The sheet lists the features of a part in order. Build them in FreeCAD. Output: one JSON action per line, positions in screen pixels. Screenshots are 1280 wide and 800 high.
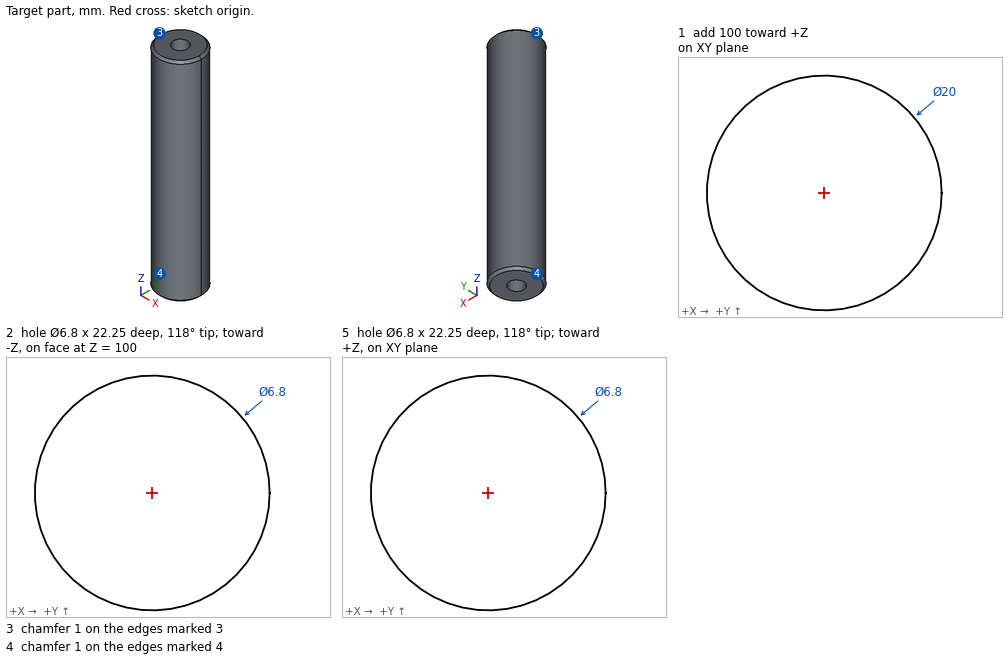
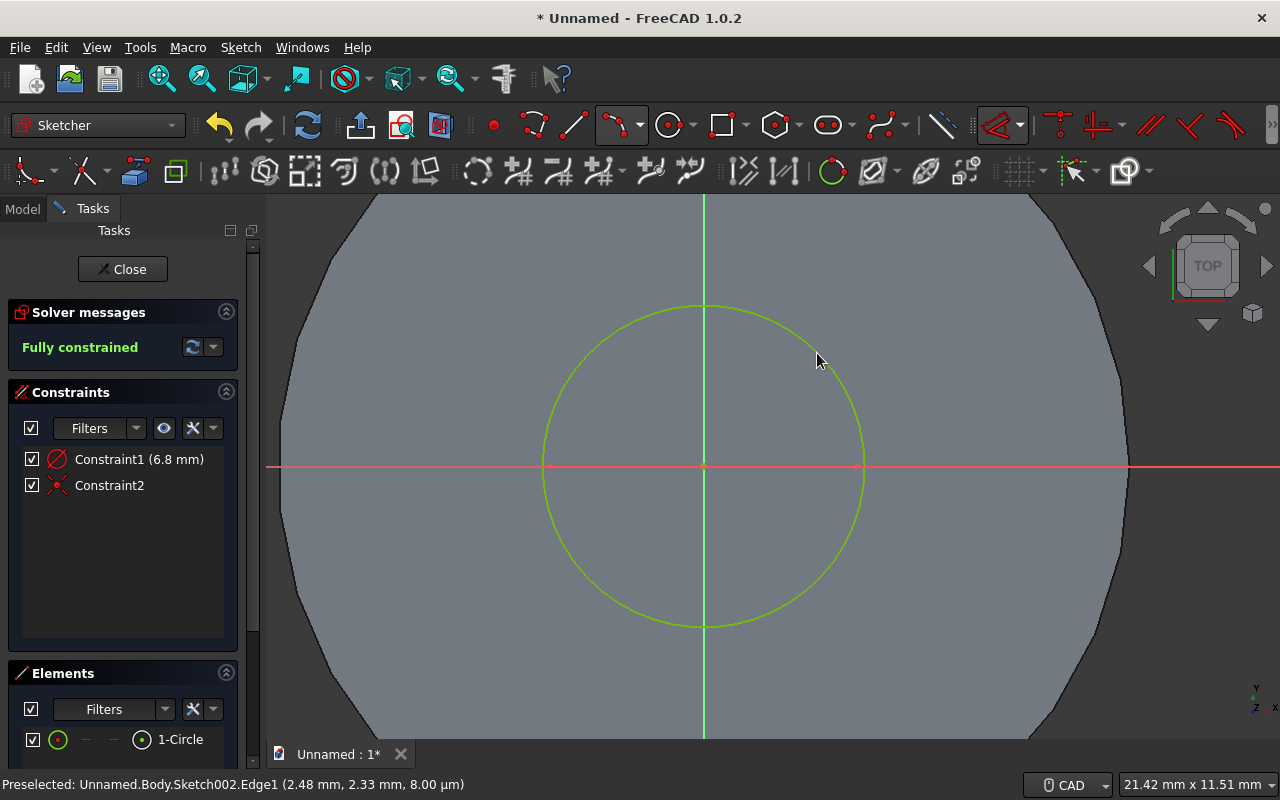
{"action": "left_click", "coordinate": [123, 269]}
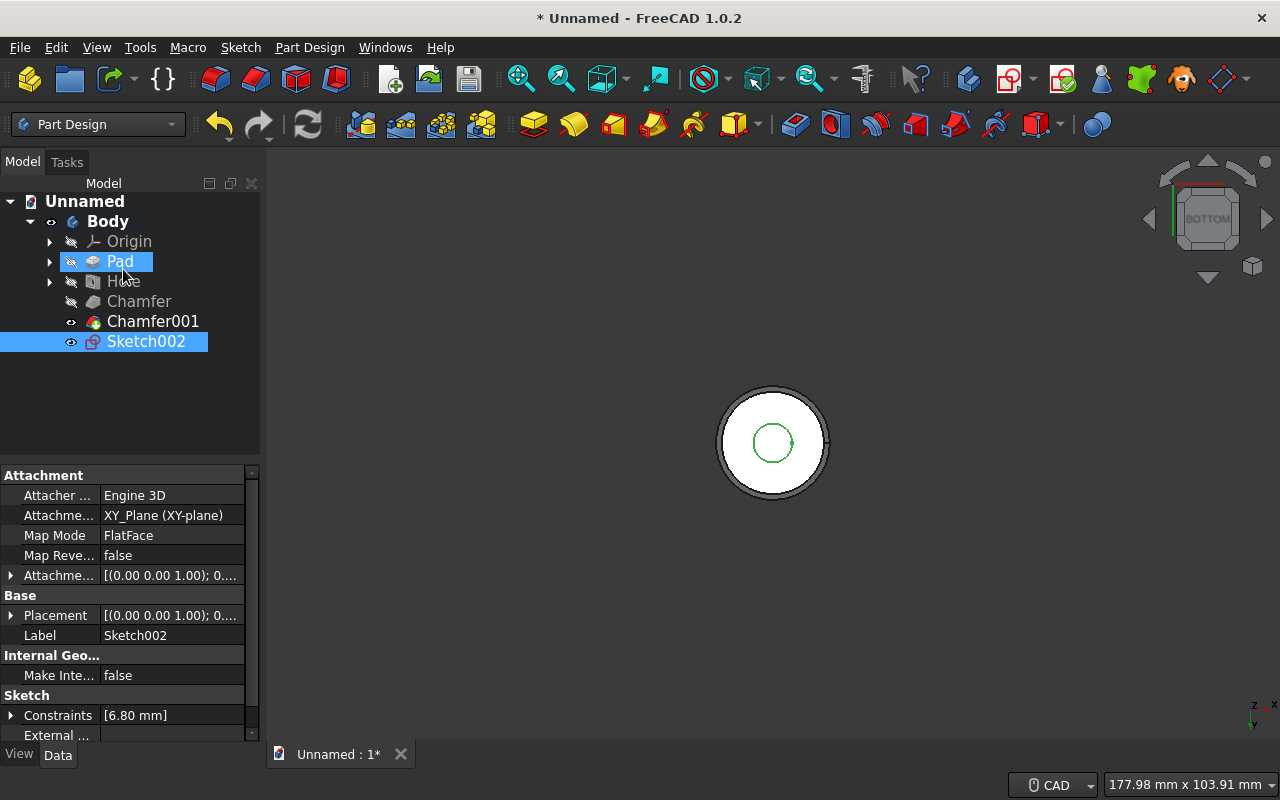
{"action": "left_click", "coordinate": [836, 124]}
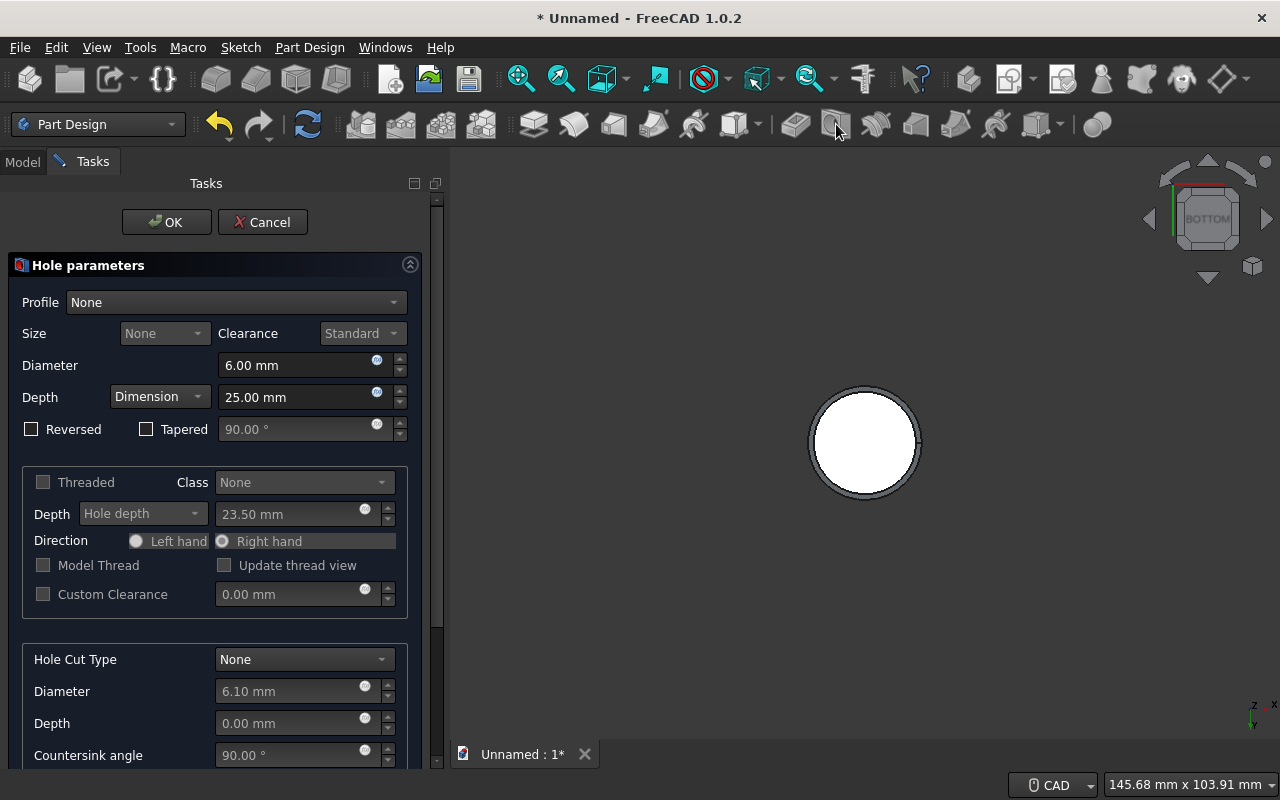
{"action": "triple_click", "coordinate": [305, 365]}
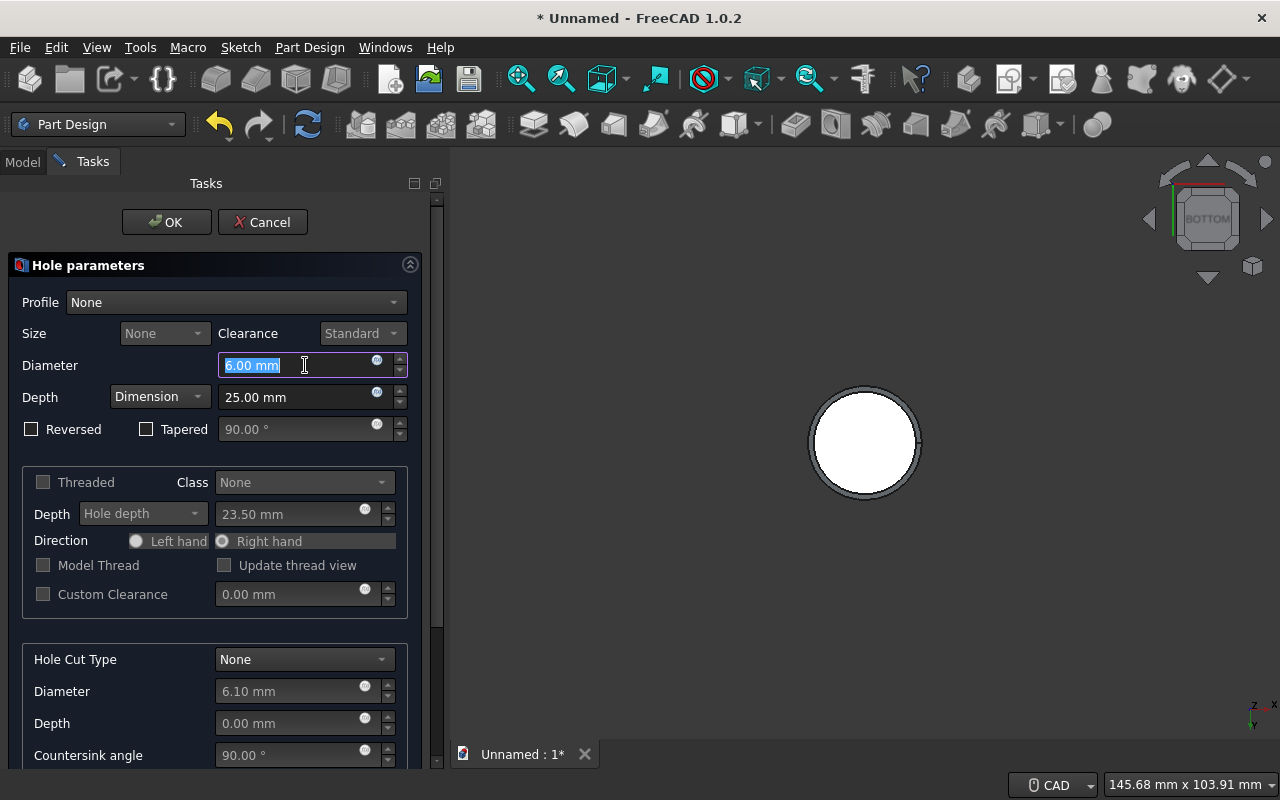
{"action": "type", "text": "6.8"}
{"action": "key", "text": "Tab"}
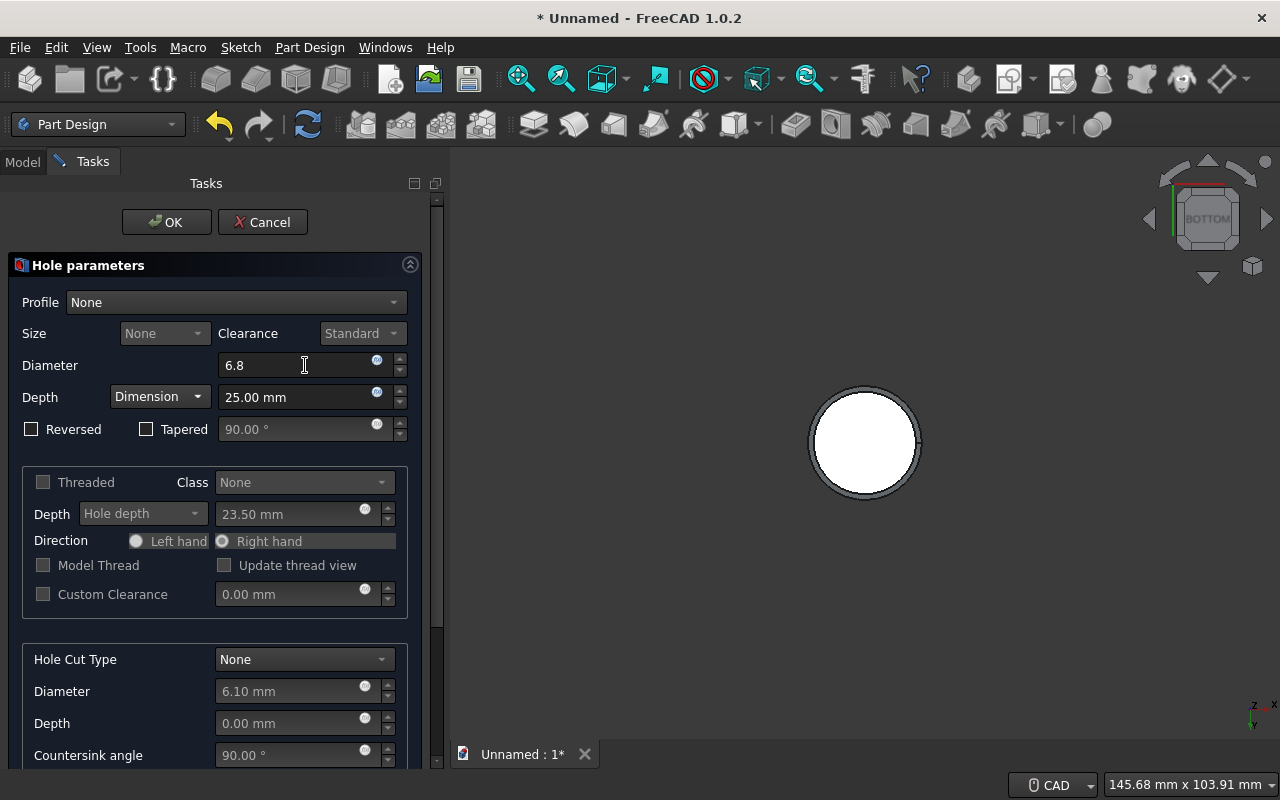
{"action": "triple_click", "coordinate": [305, 397]}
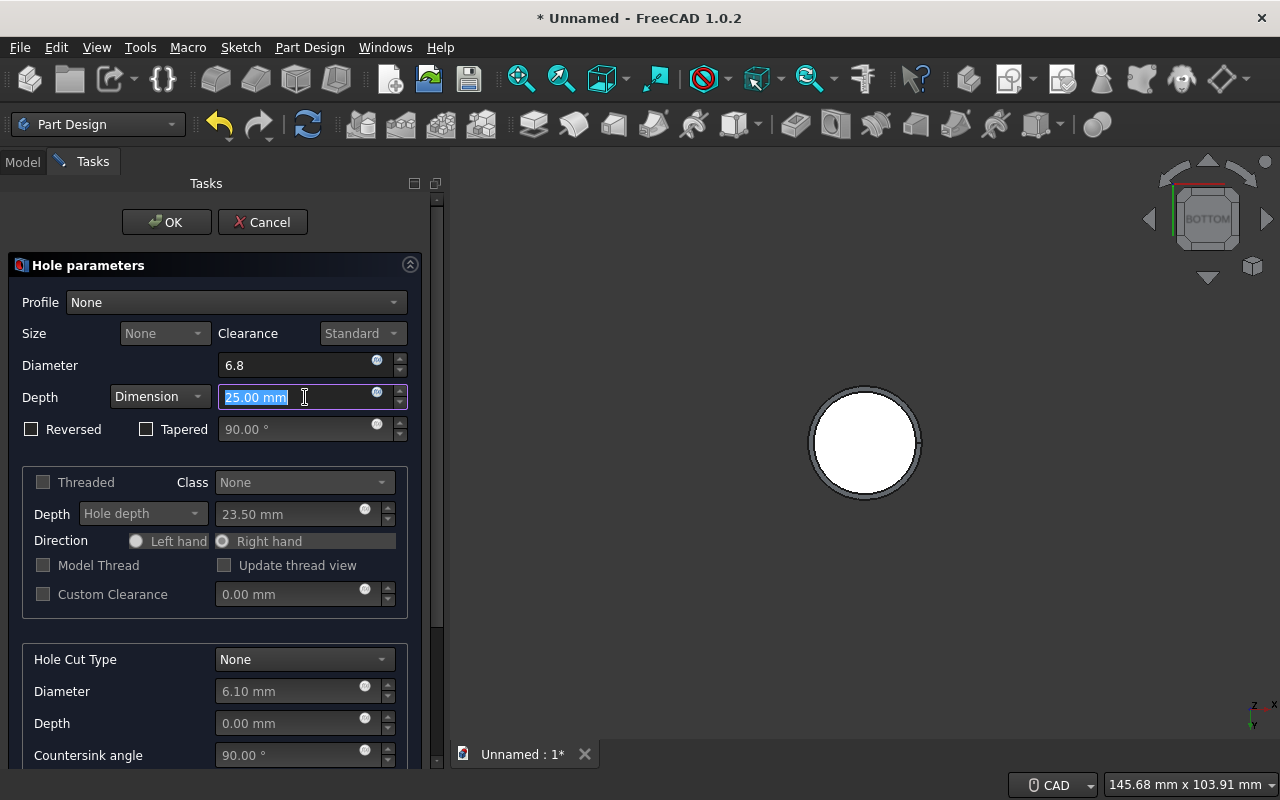
{"action": "type", "text": "22.25"}
{"action": "key", "text": "Tab"}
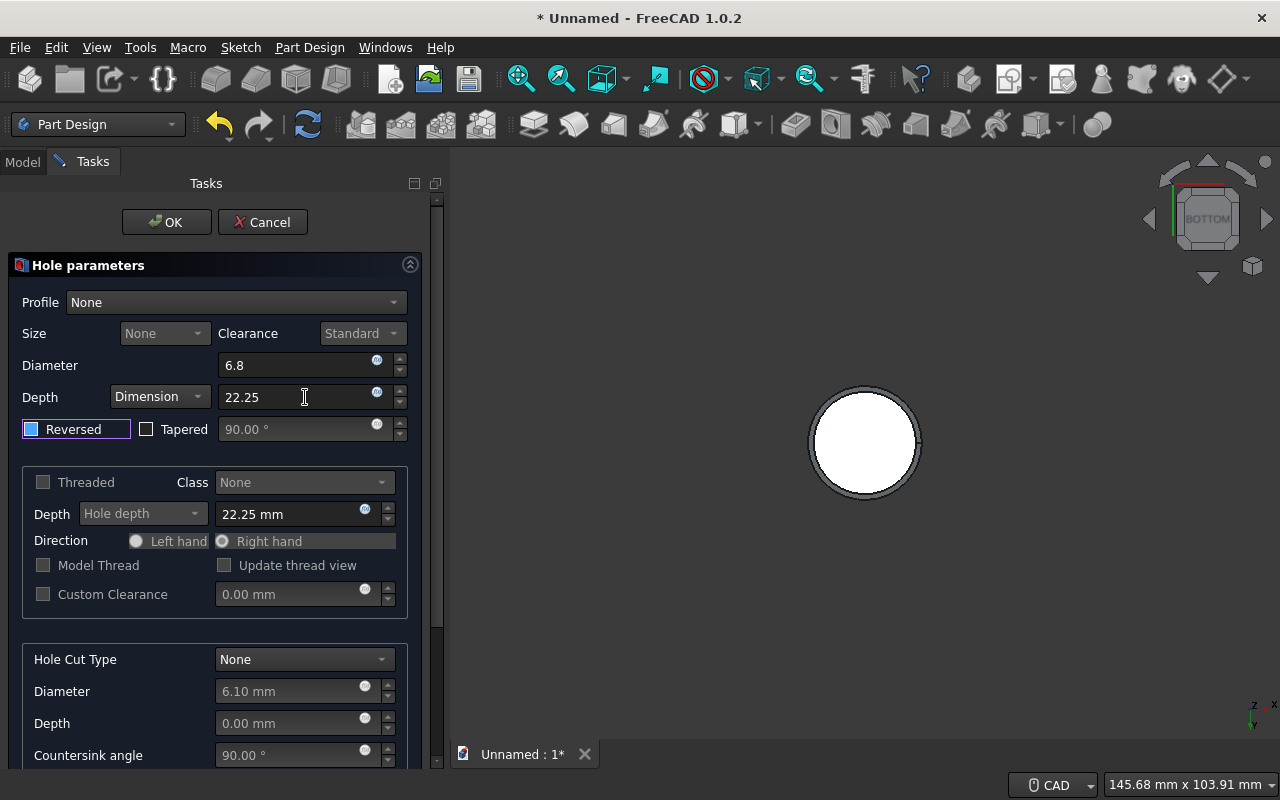
{"action": "left_click", "coordinate": [30, 429]}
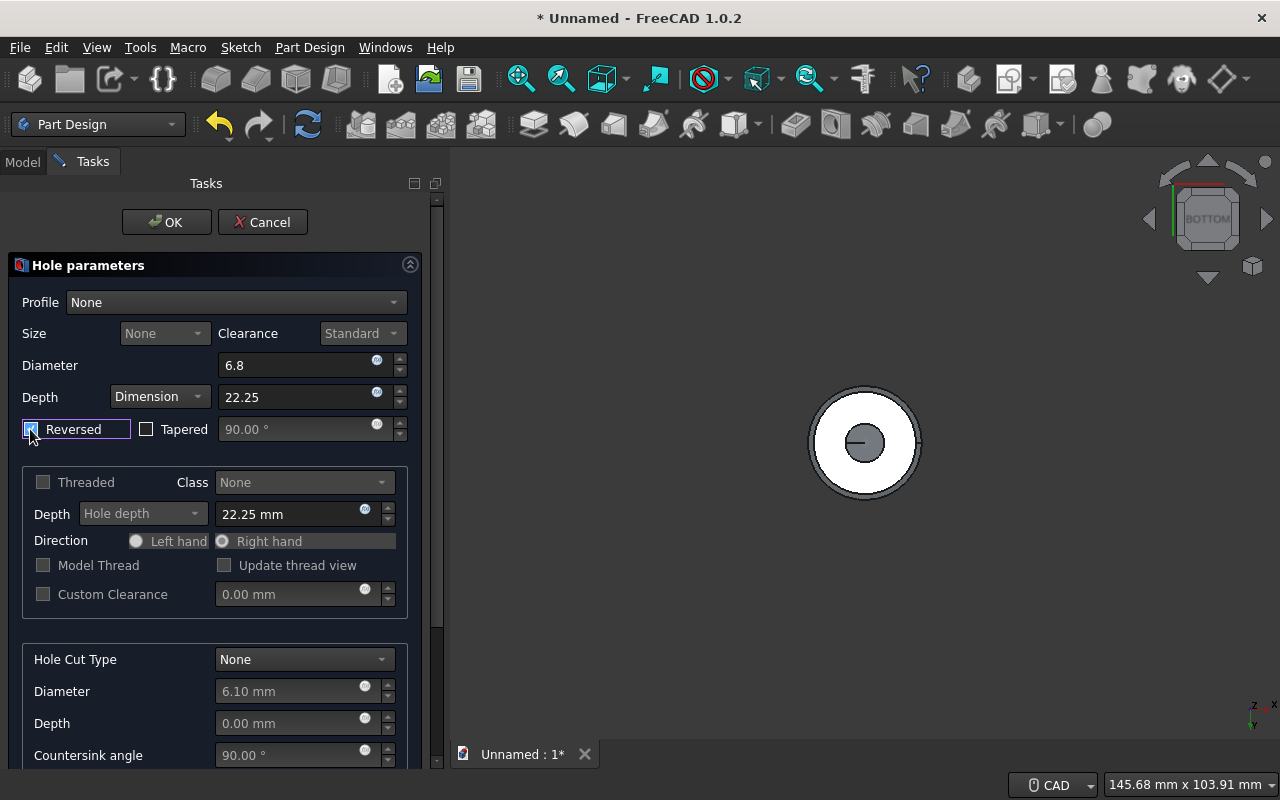
{"action": "left_click", "coordinate": [167, 222]}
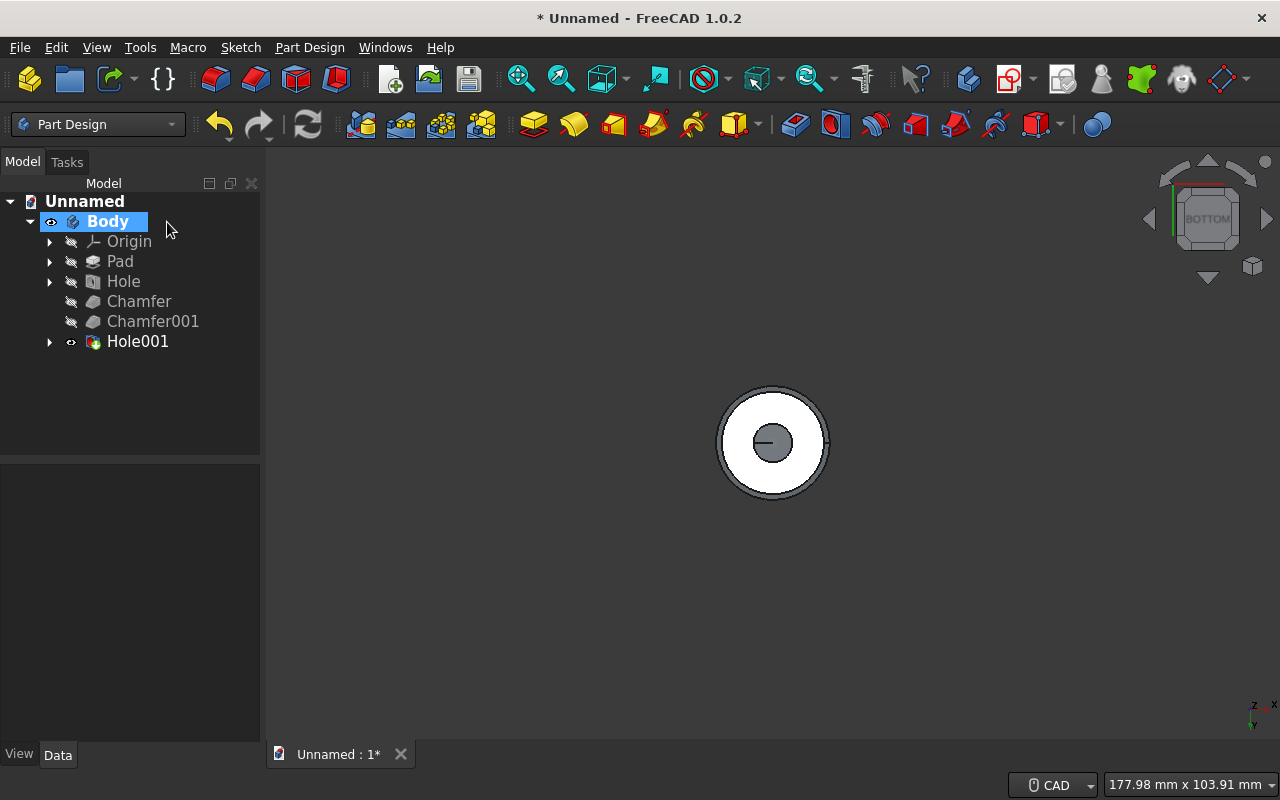
{"action": "key", "text": "0"}